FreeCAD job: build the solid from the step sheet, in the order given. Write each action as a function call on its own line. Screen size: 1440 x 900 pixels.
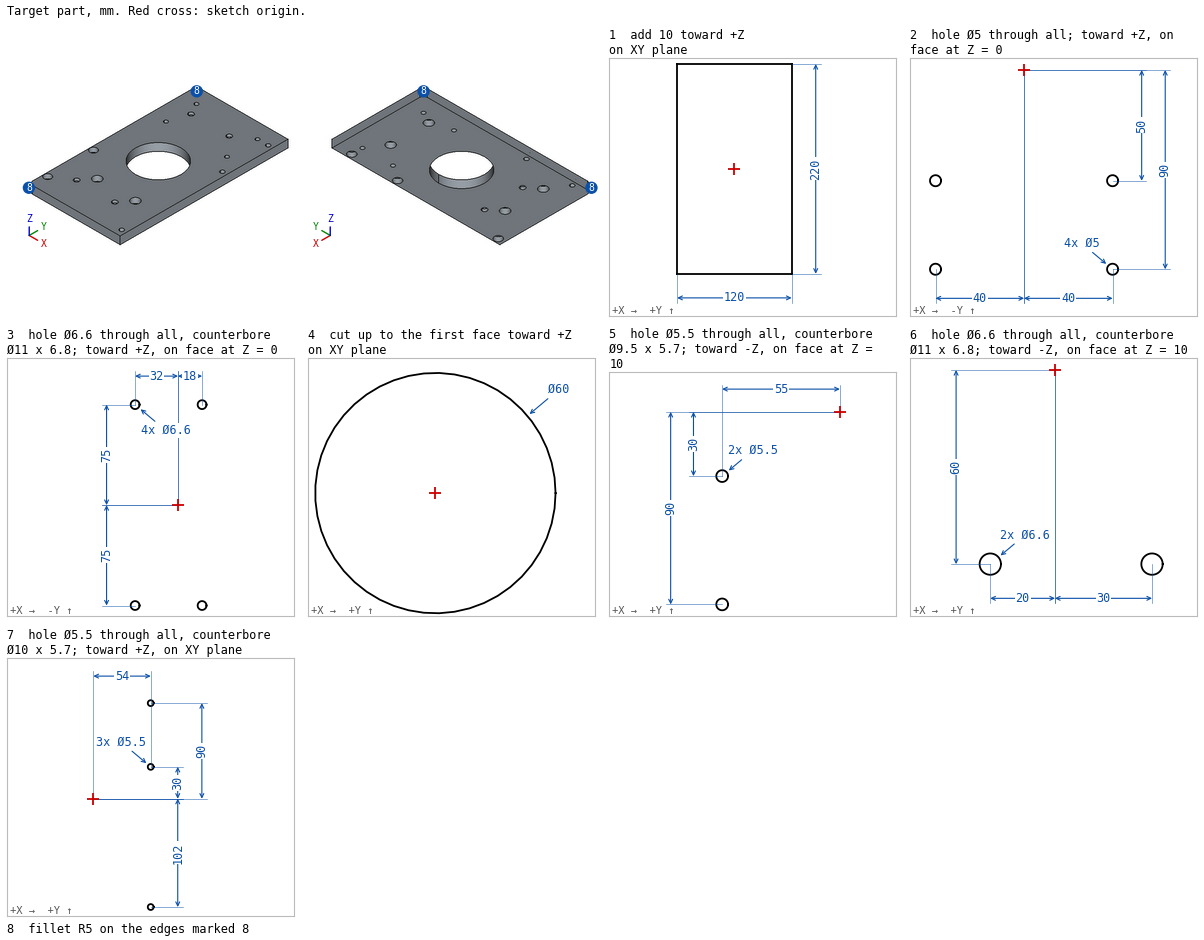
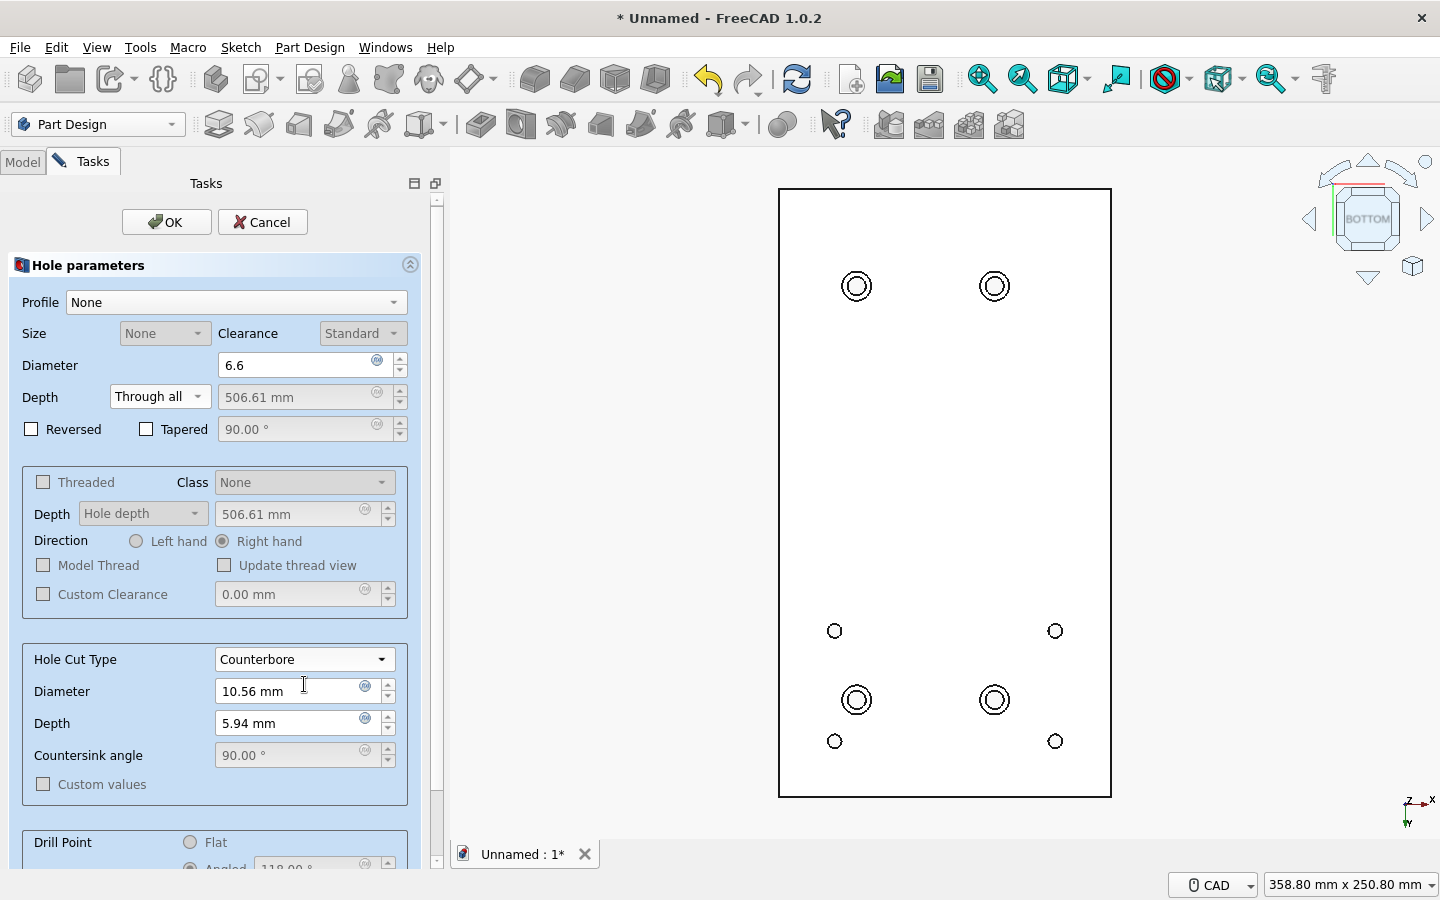
triple_click(298, 691)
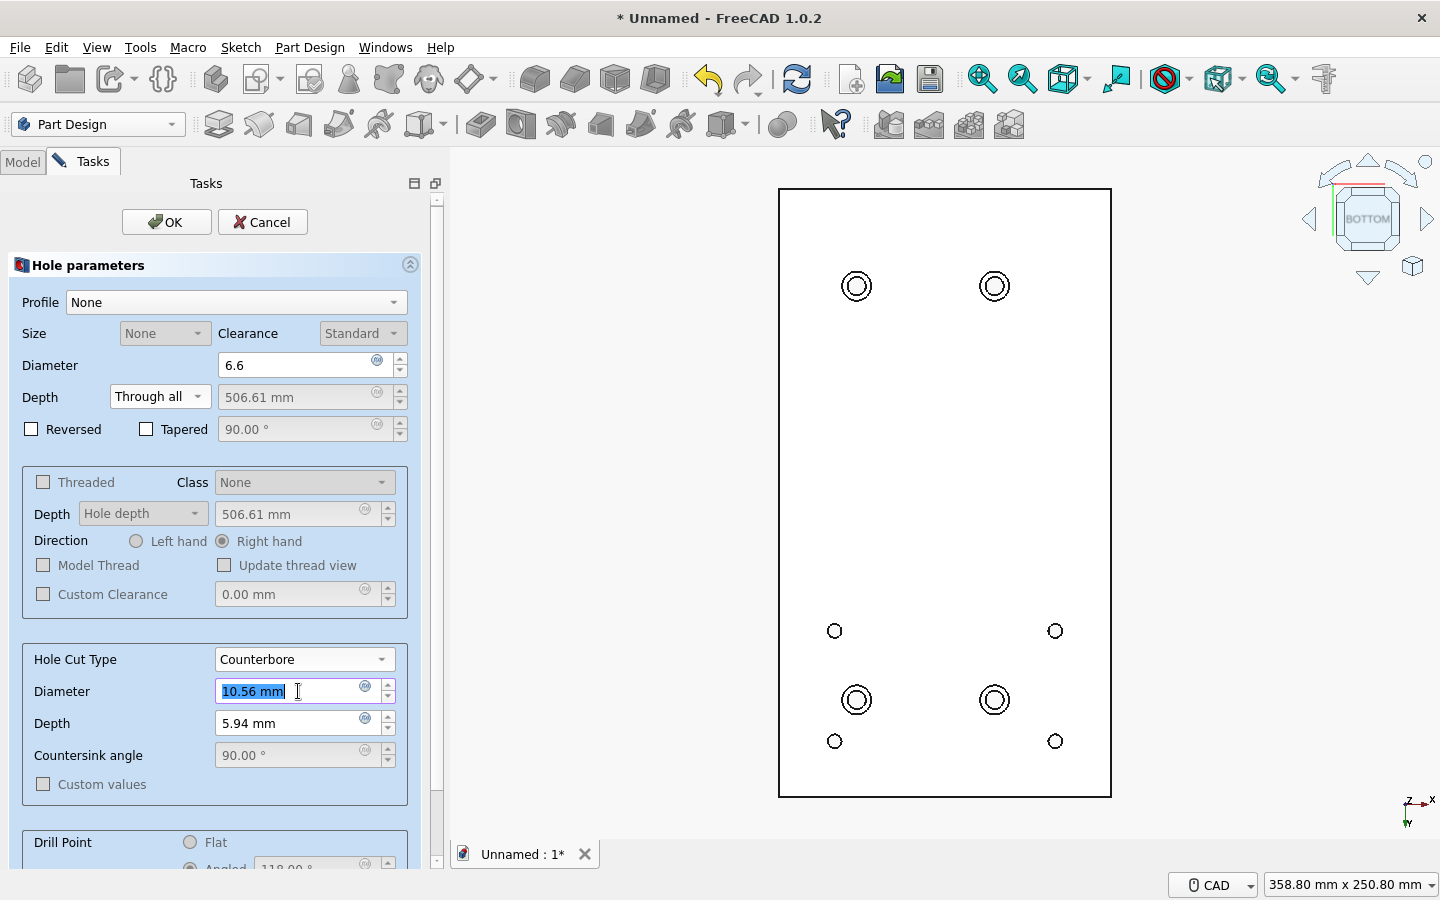
text(11)
key(Tab)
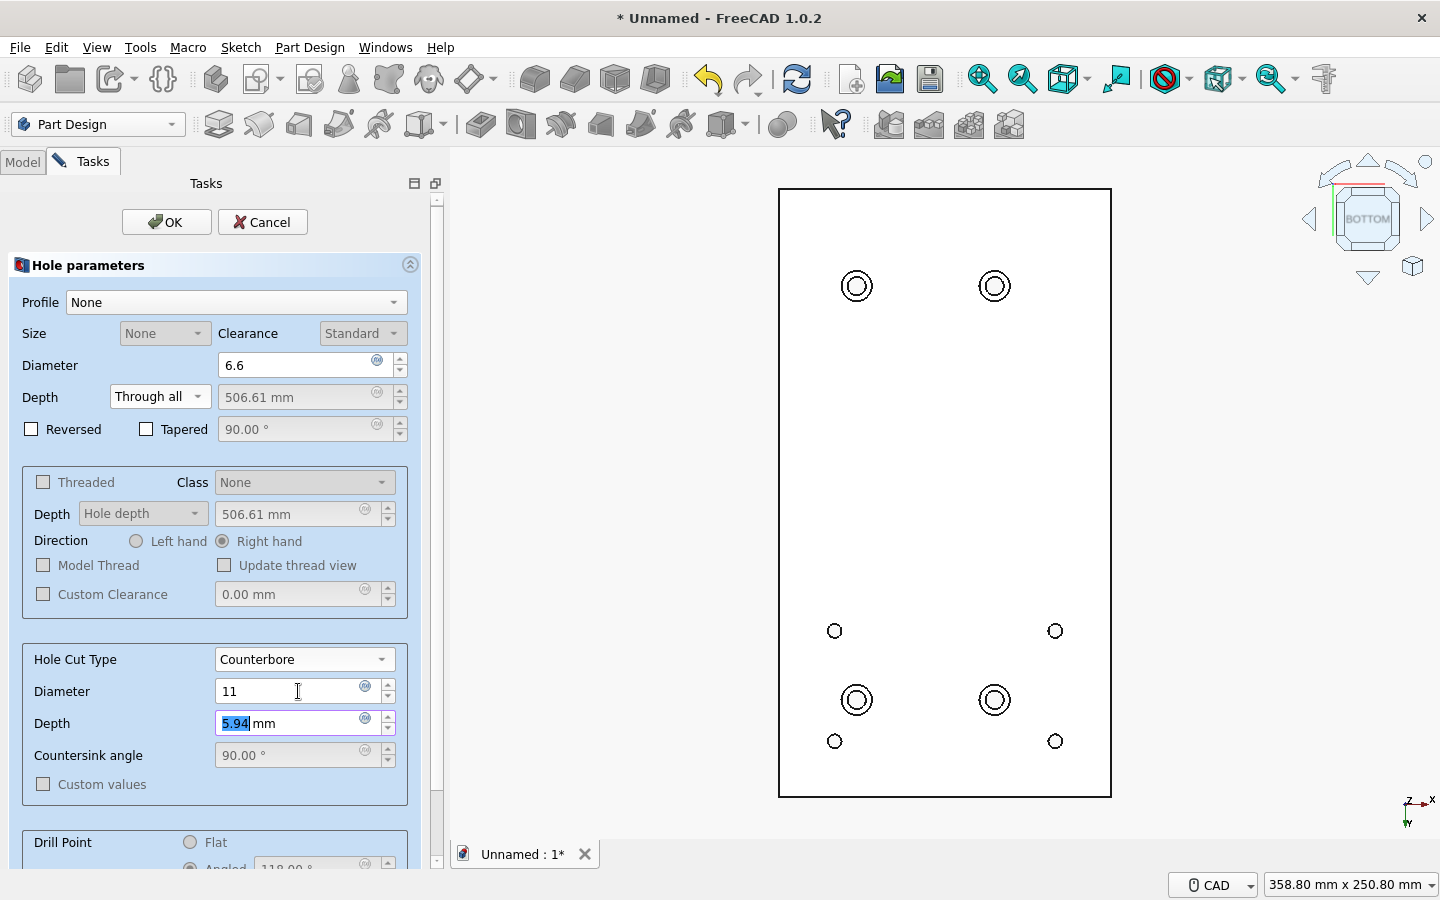
text(6.8)
key(Tab)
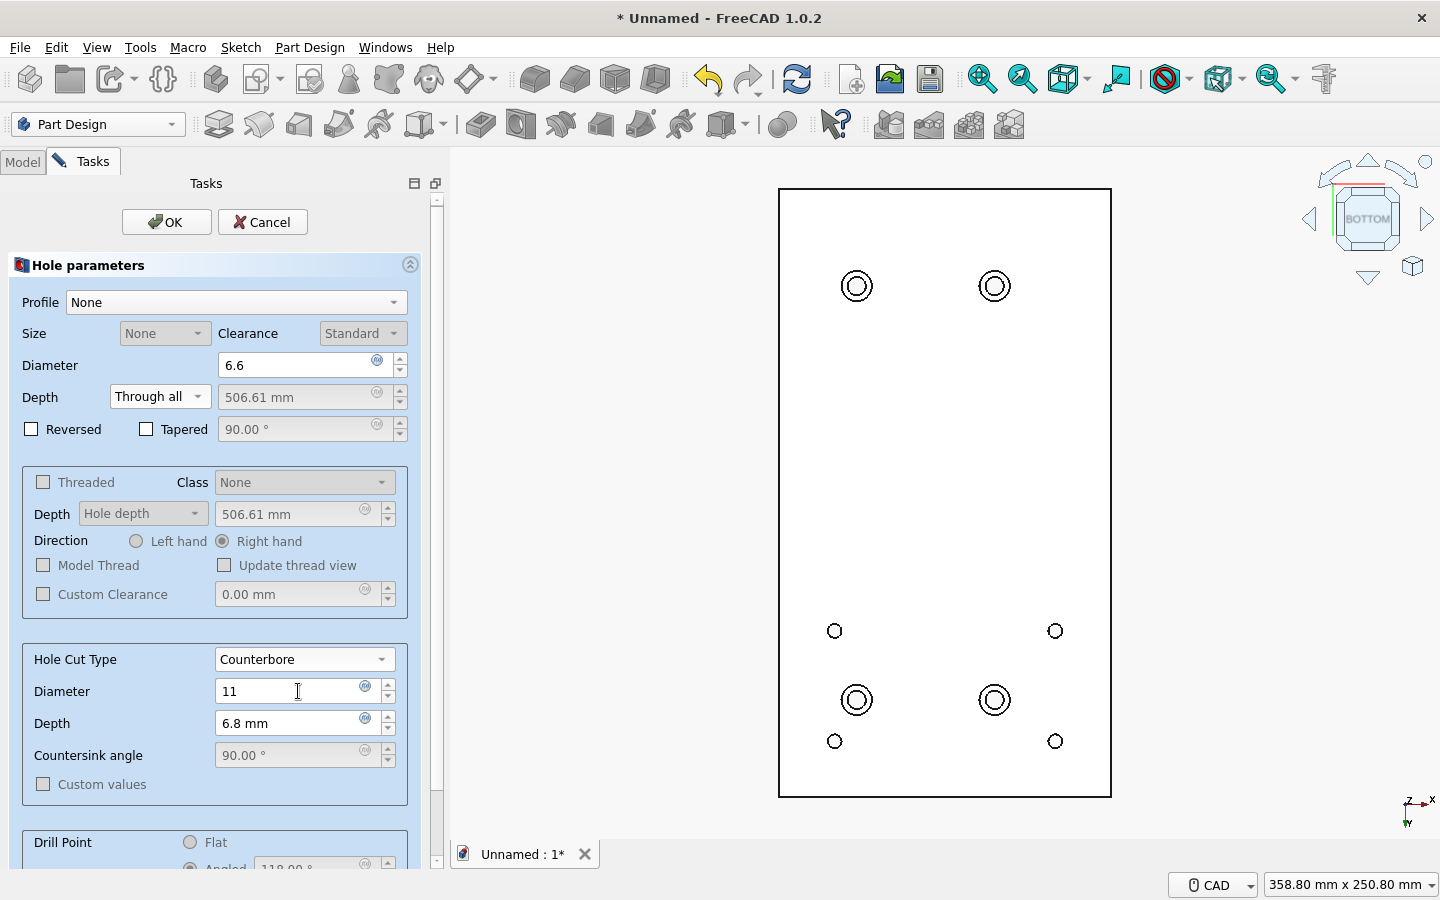
click(167, 222)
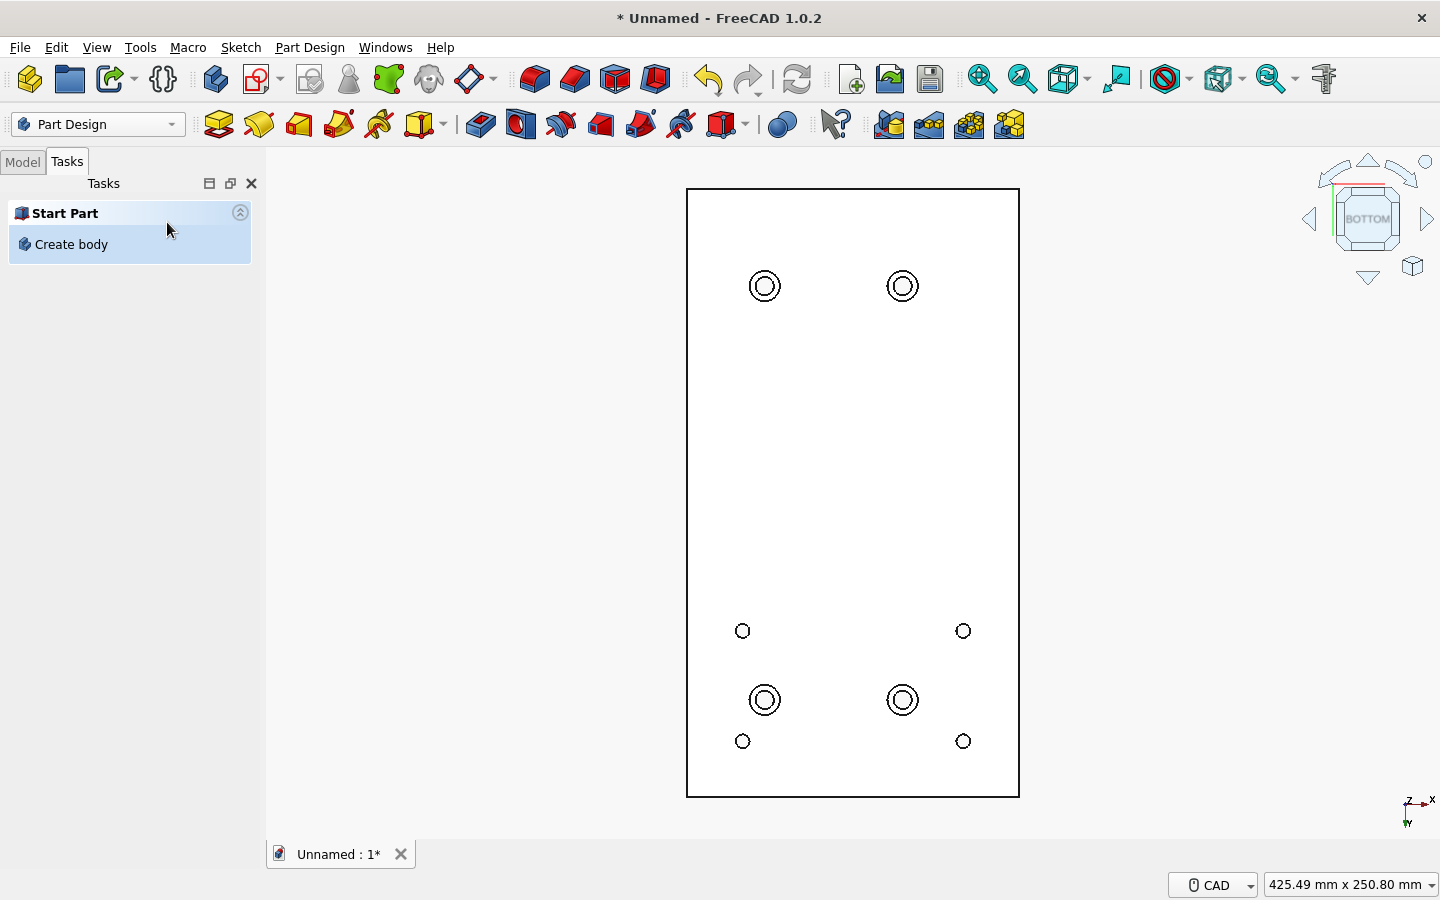
click(256, 80)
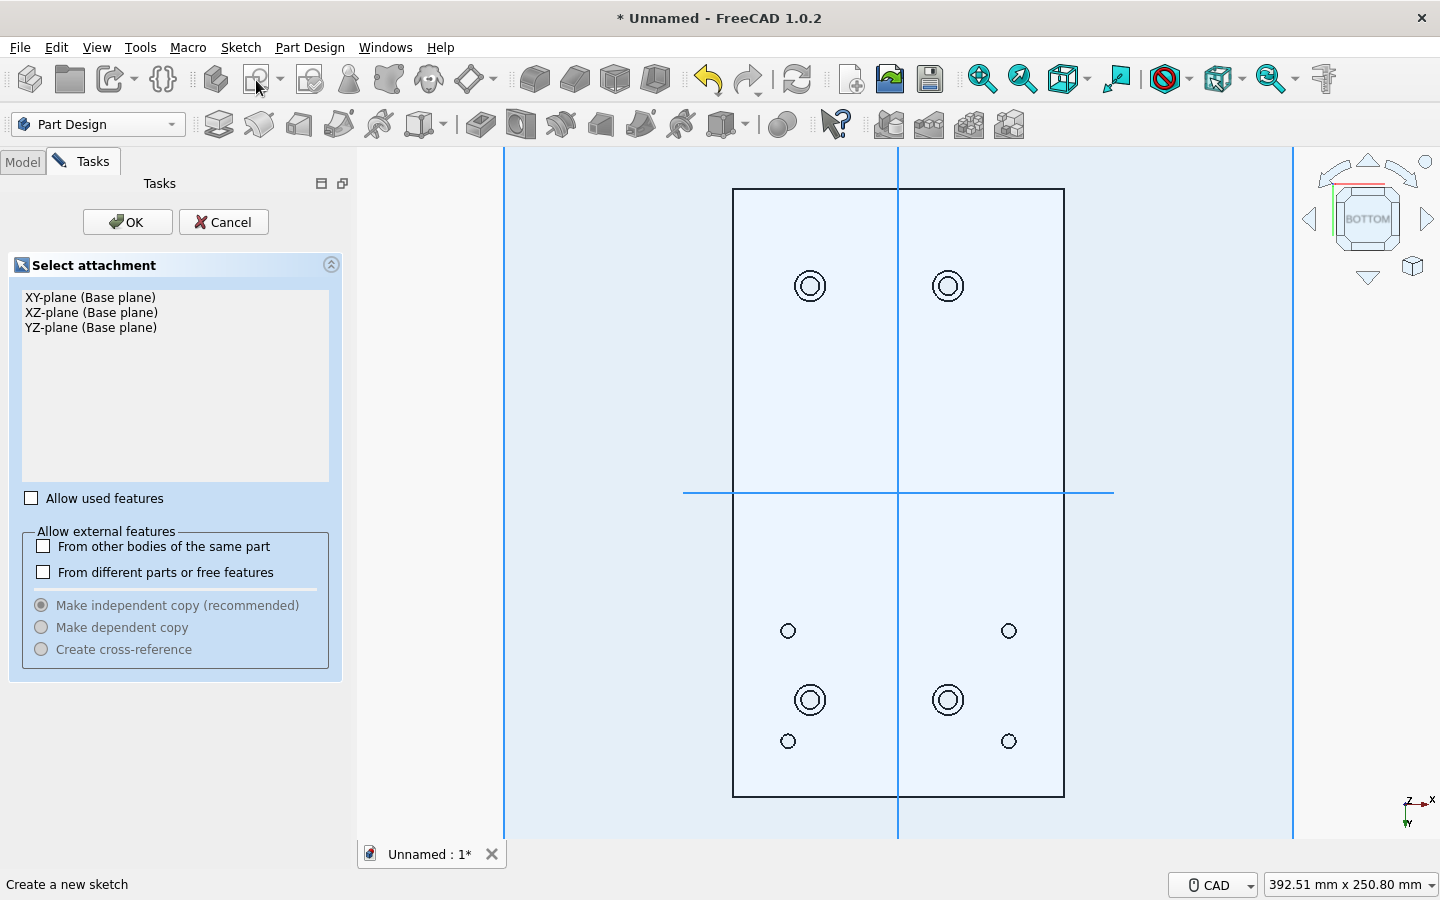
click(82, 298)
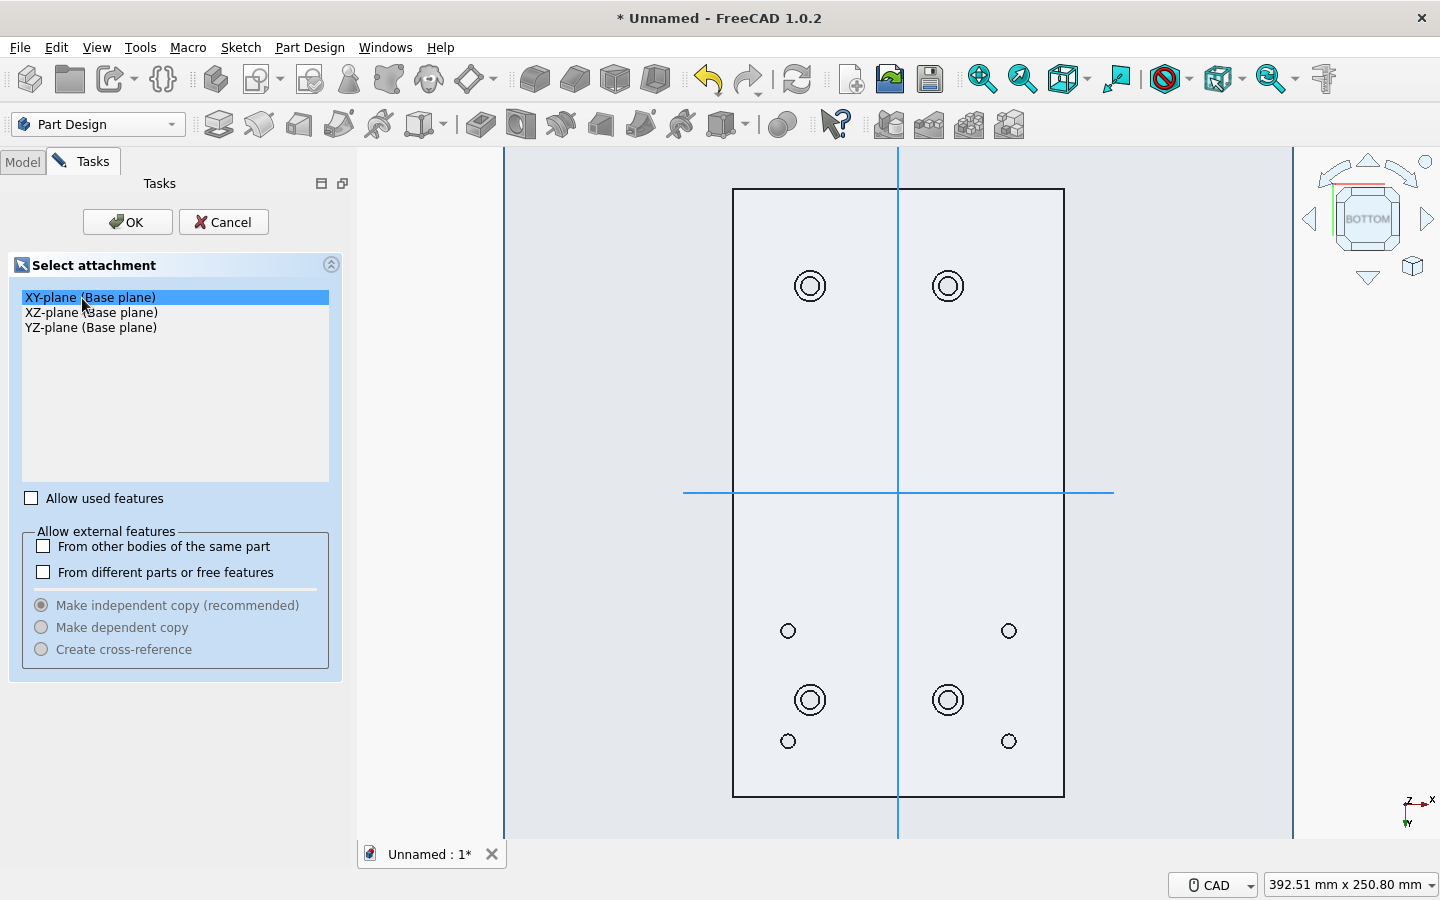
click(128, 222)